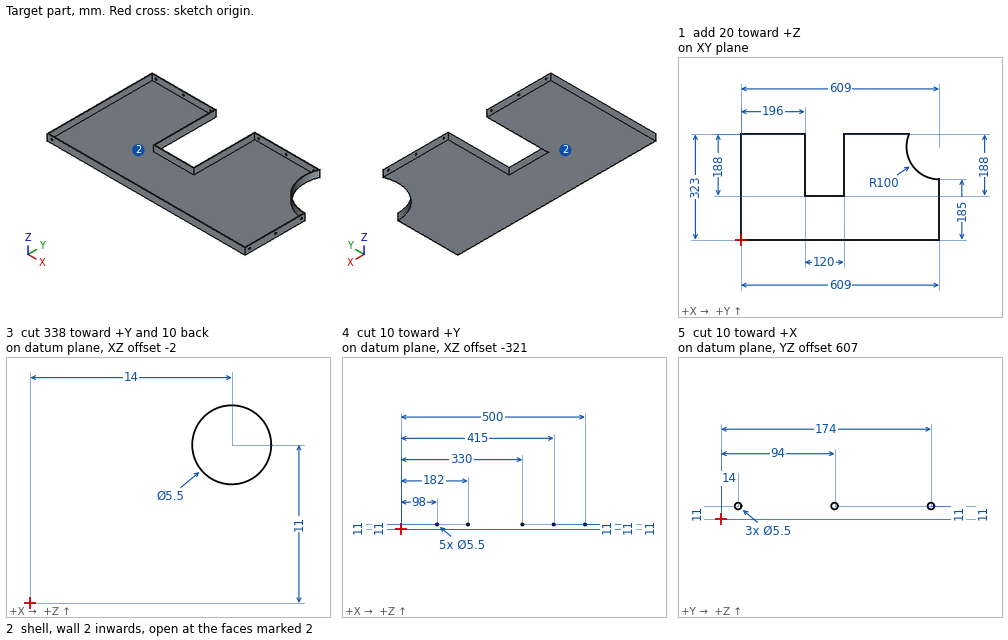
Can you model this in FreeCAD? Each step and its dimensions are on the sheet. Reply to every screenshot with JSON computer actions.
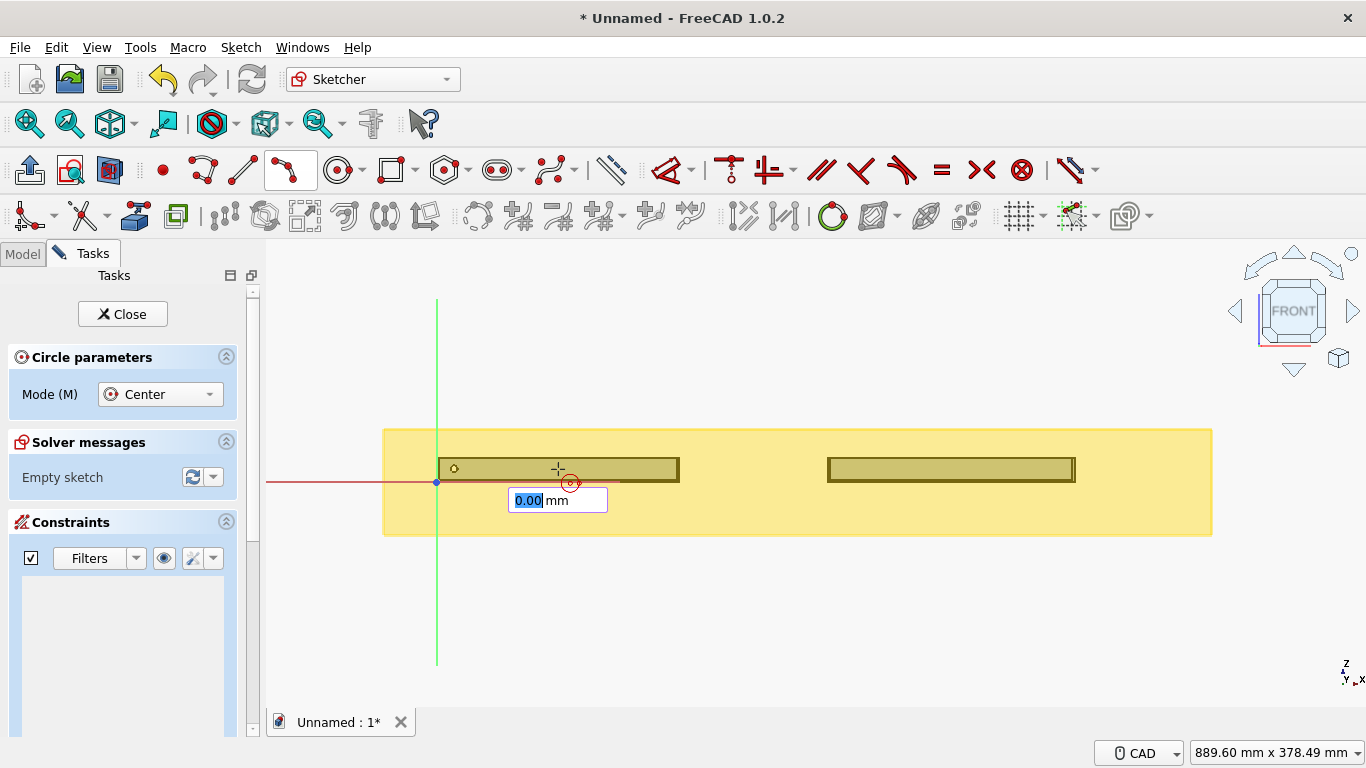
{"action": "scroll", "coordinate": [560, 466], "scroll_direction": "up", "scroll_amount": 8}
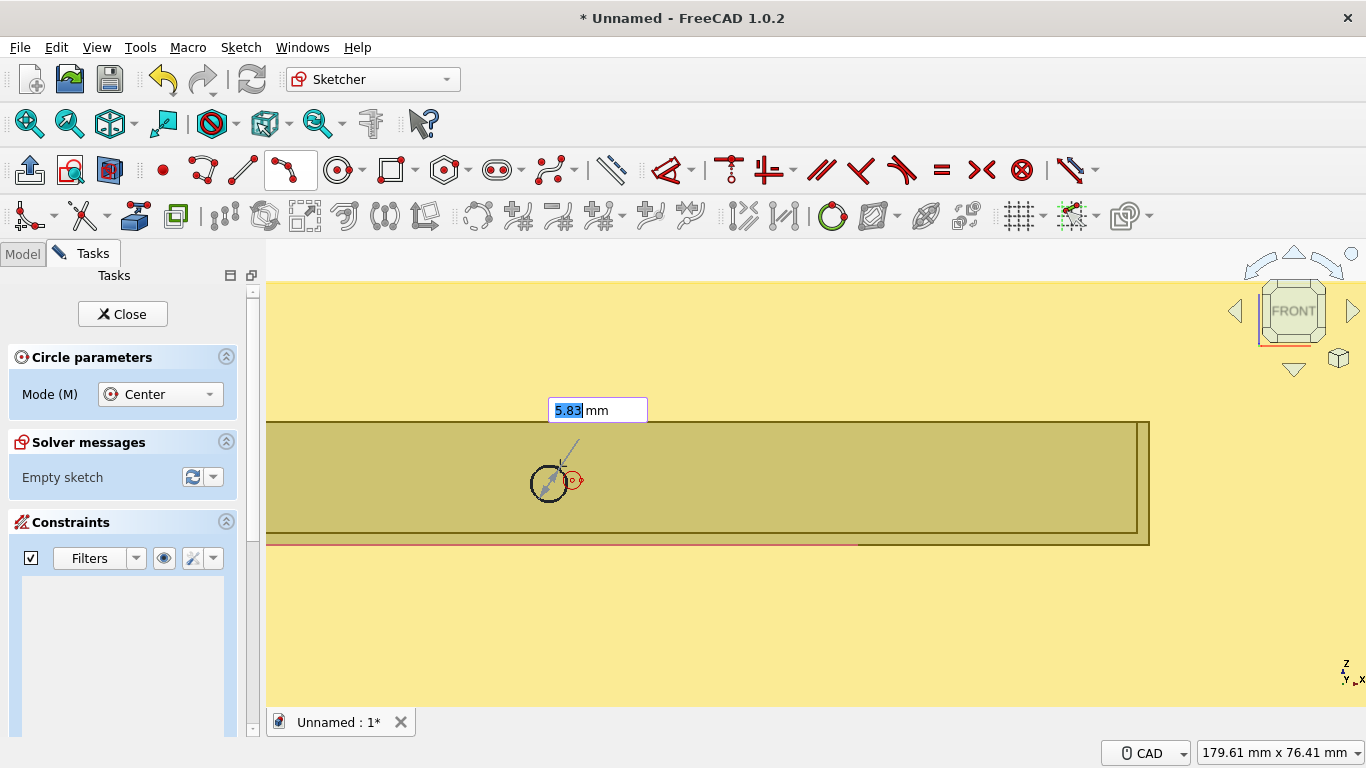
{"action": "left_click", "coordinate": [561, 466]}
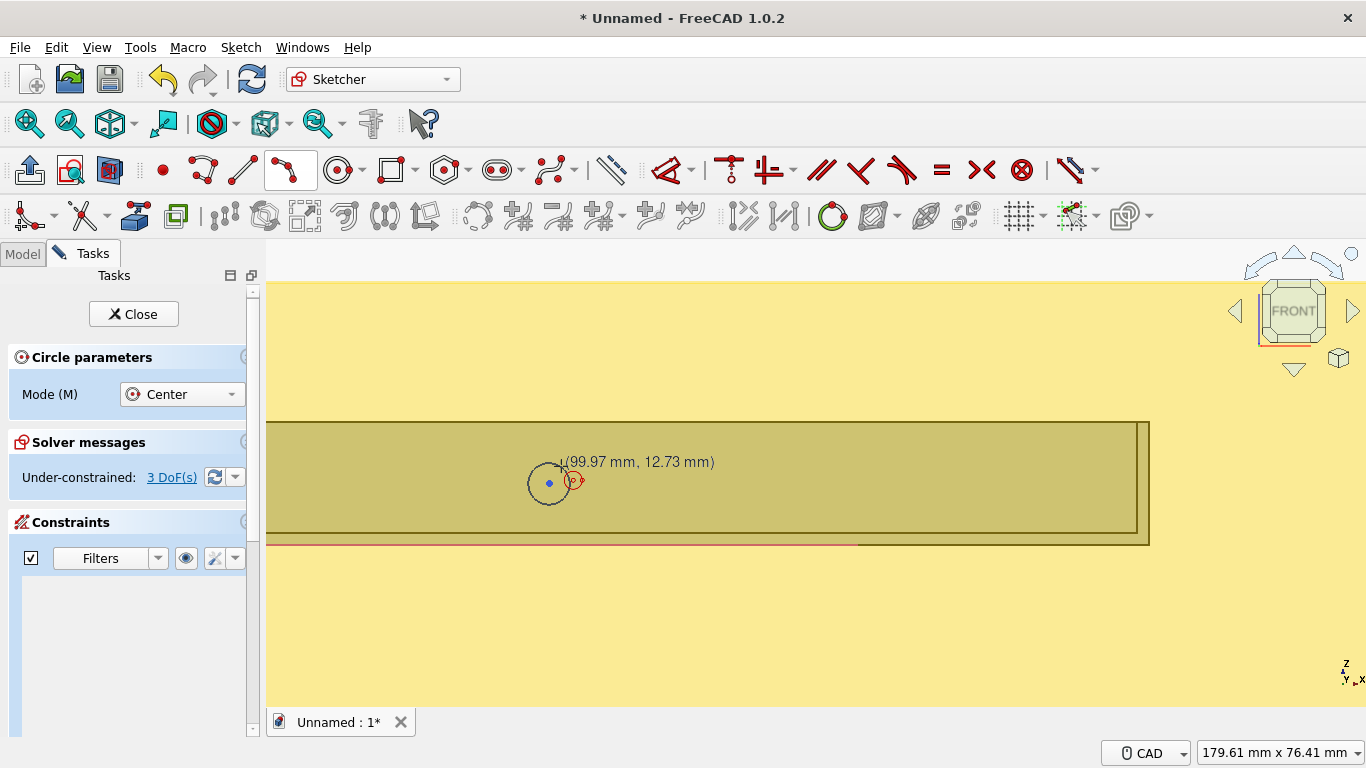
{"action": "scroll", "coordinate": [1063, 478], "scroll_direction": "up", "scroll_amount": 2}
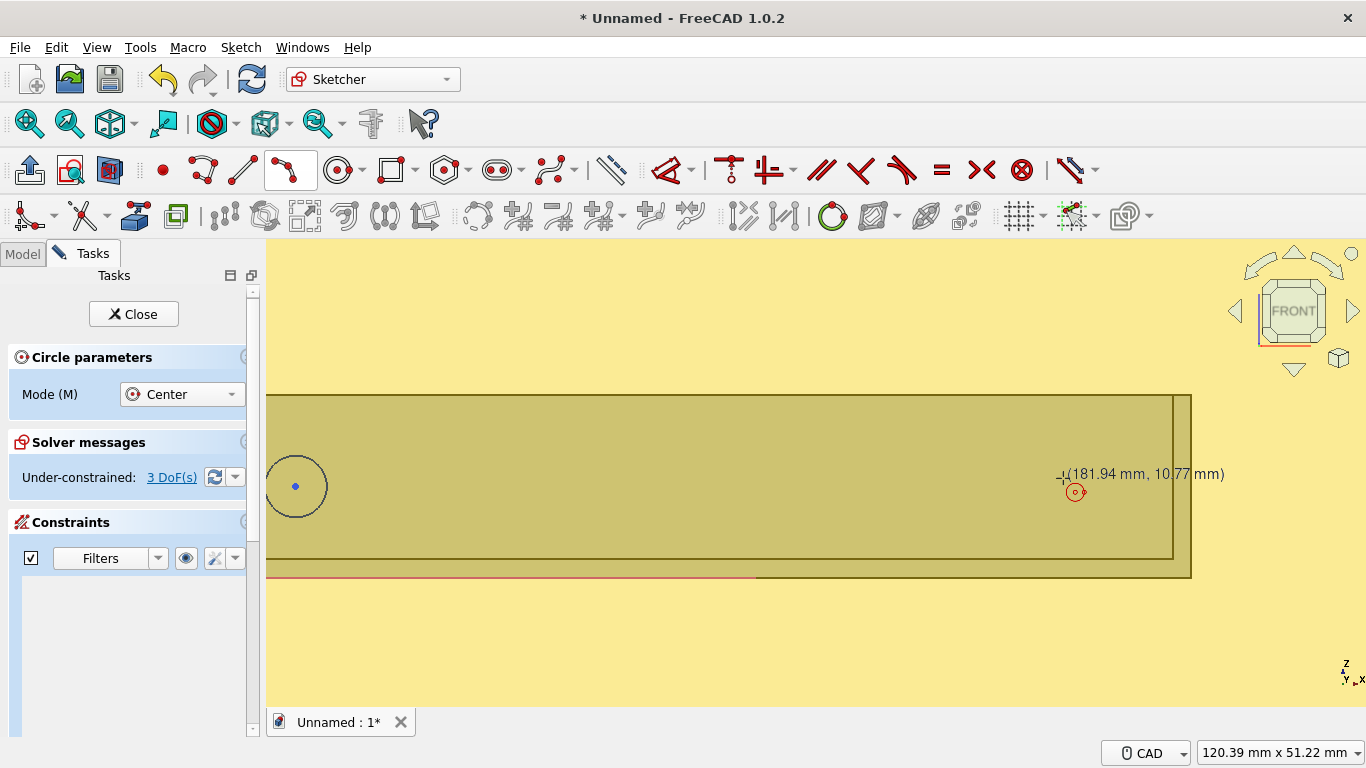
{"action": "scroll", "coordinate": [599, 466], "scroll_direction": "down", "scroll_amount": 10}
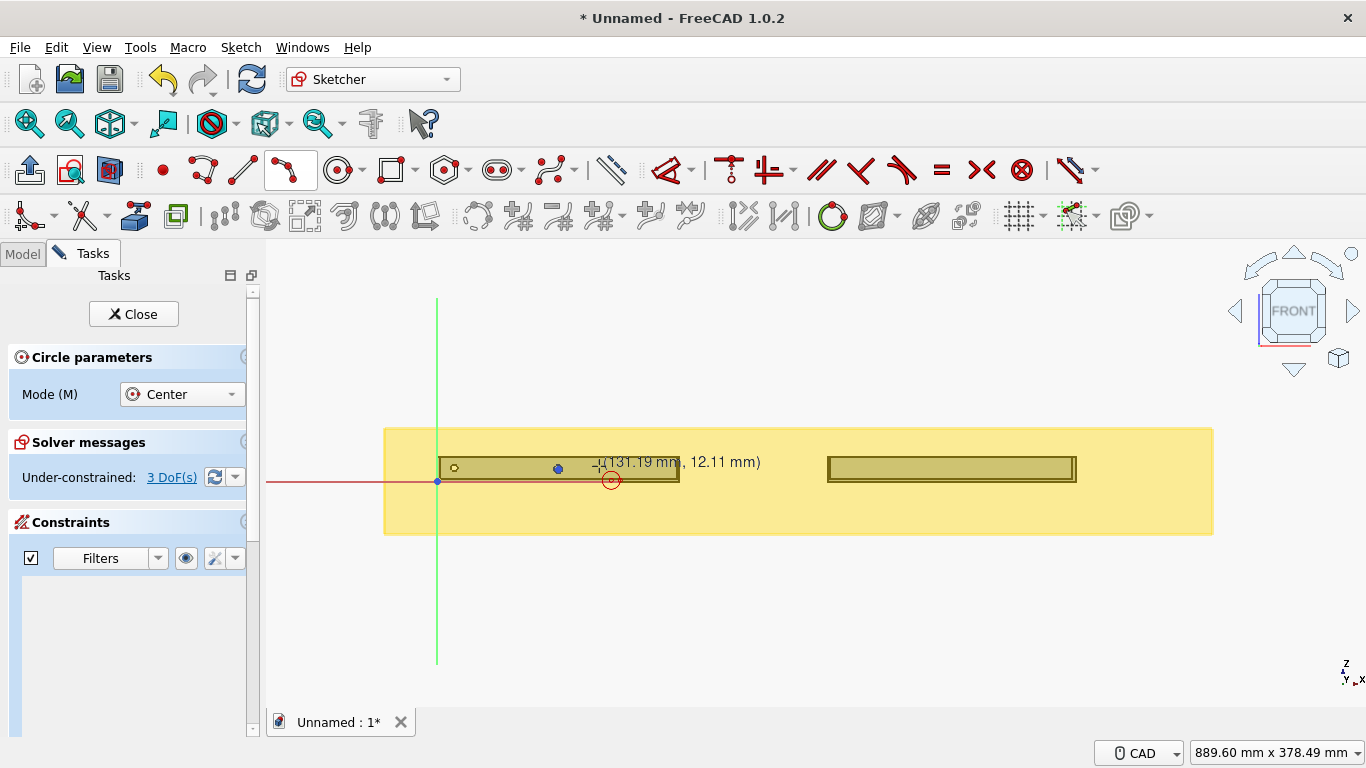
{"action": "left_click", "coordinate": [662, 468]}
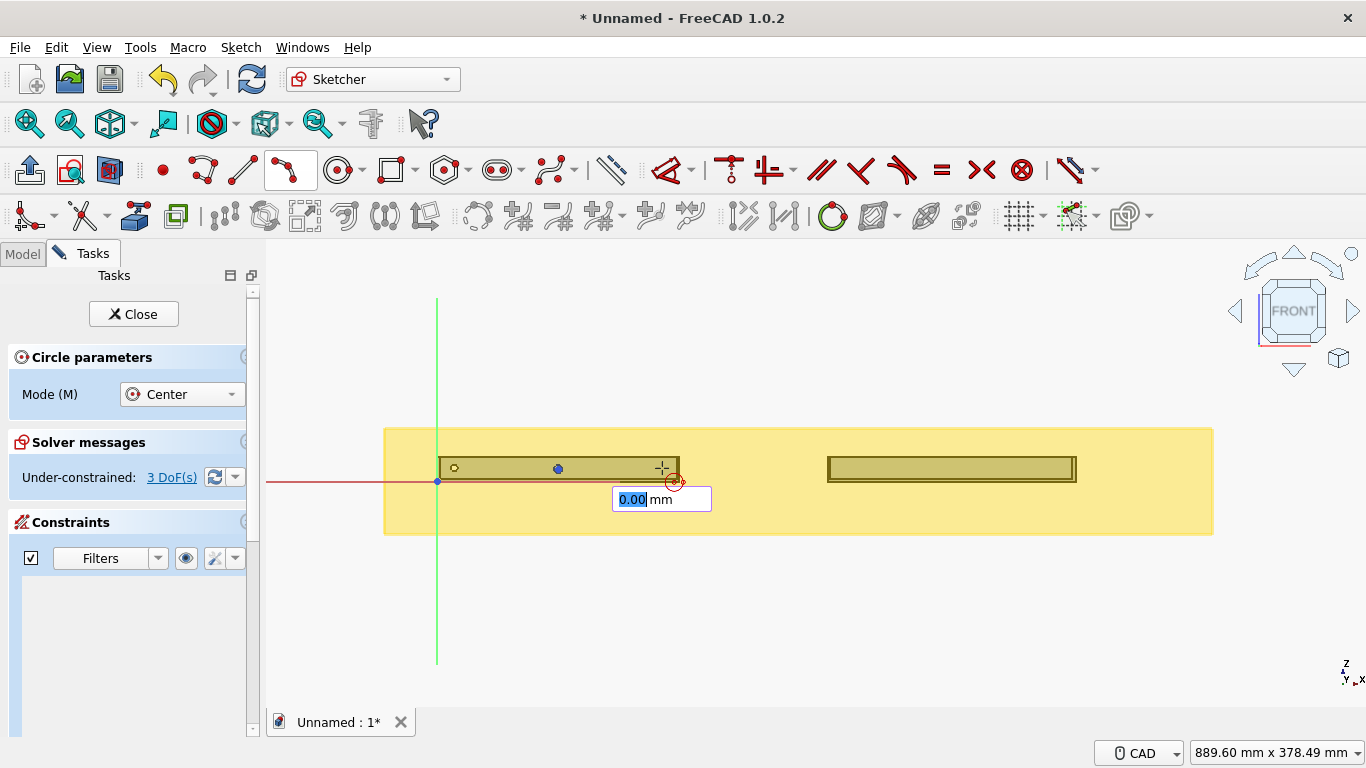
{"action": "scroll", "coordinate": [664, 466], "scroll_direction": "up", "scroll_amount": 8}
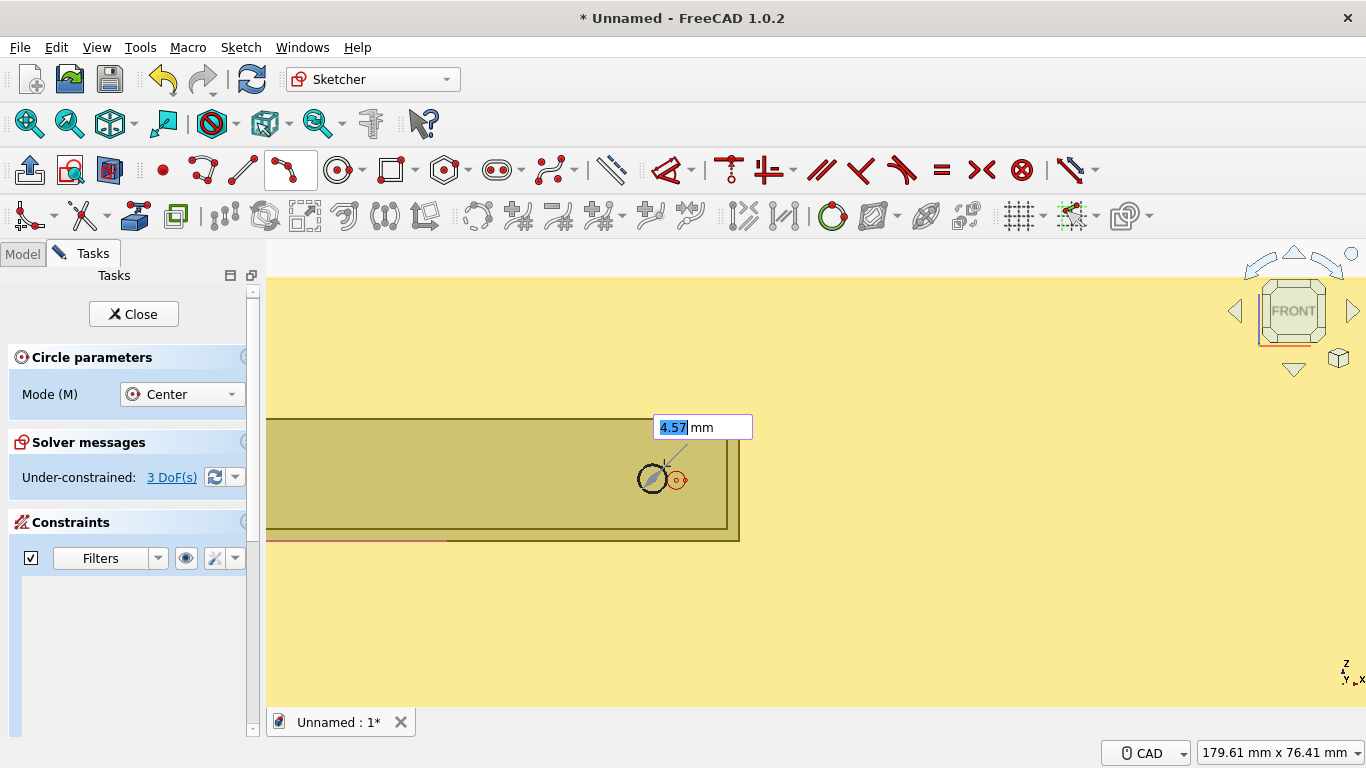
{"action": "left_click", "coordinate": [665, 462]}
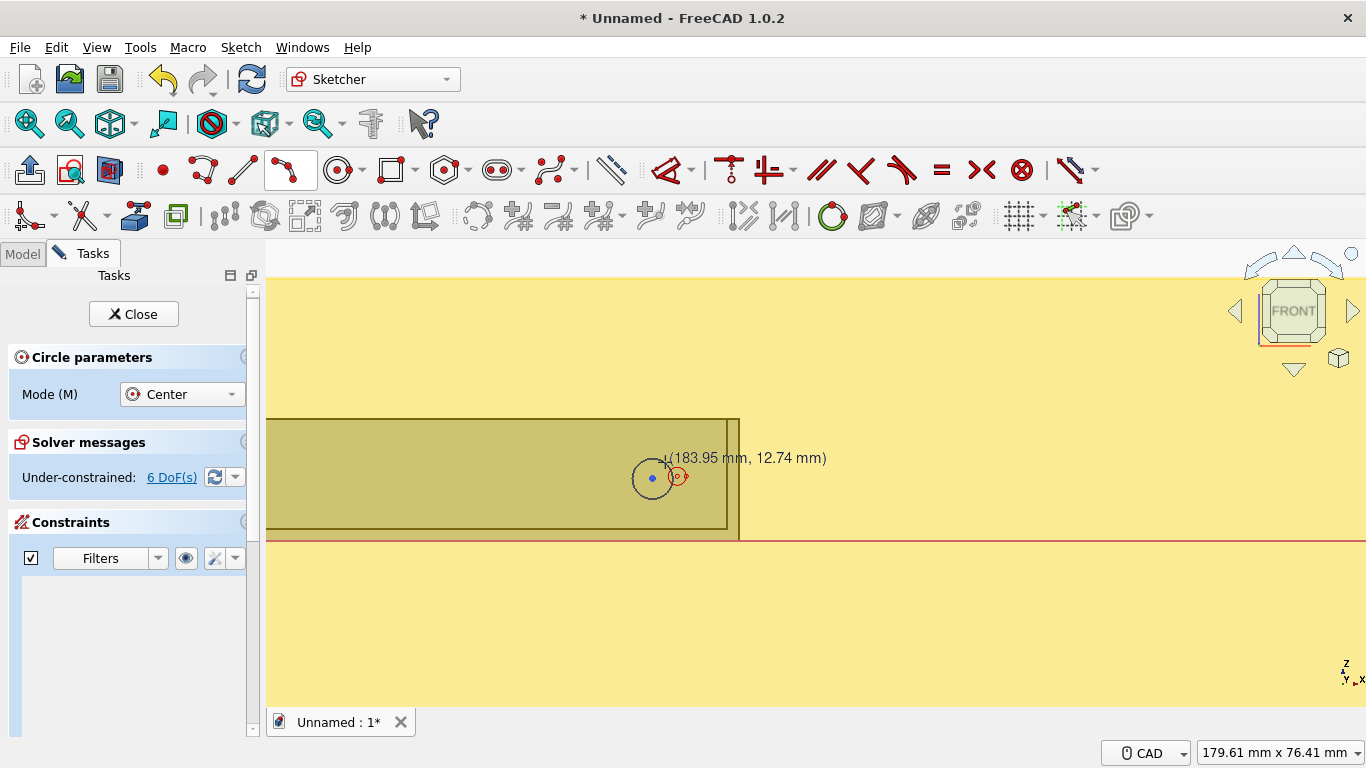
{"action": "scroll", "coordinate": [664, 466], "scroll_direction": "down", "scroll_amount": 8}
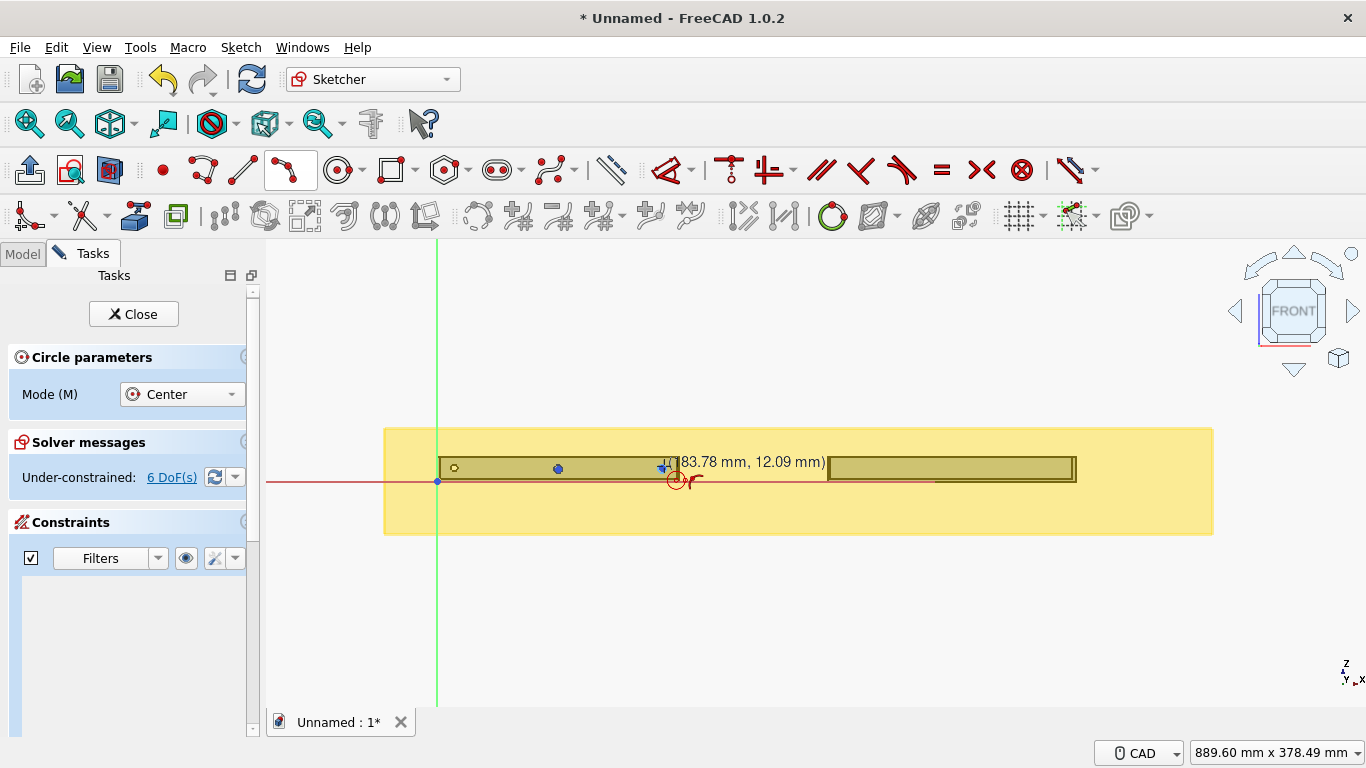
{"action": "scroll", "coordinate": [845, 468], "scroll_direction": "up", "scroll_amount": 10}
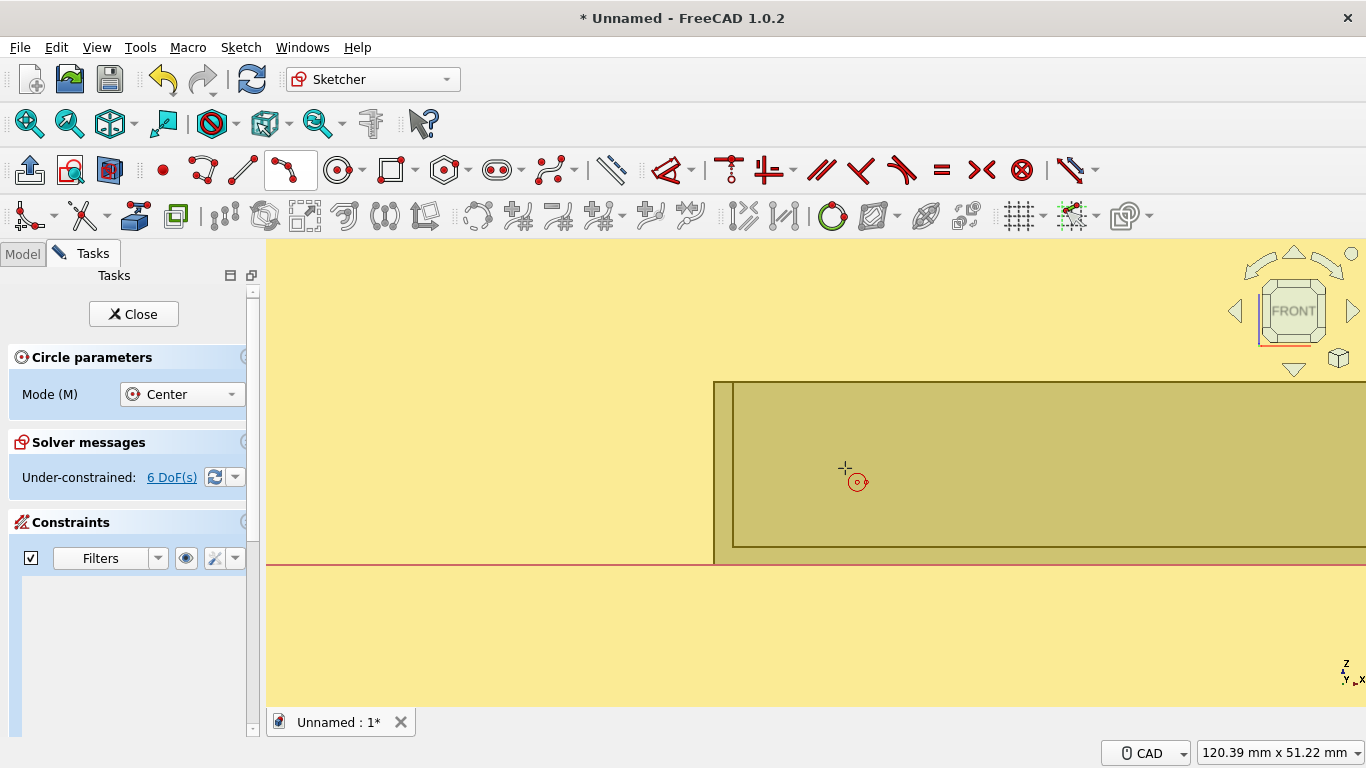
{"action": "scroll", "coordinate": [845, 468], "scroll_direction": "down", "scroll_amount": 10}